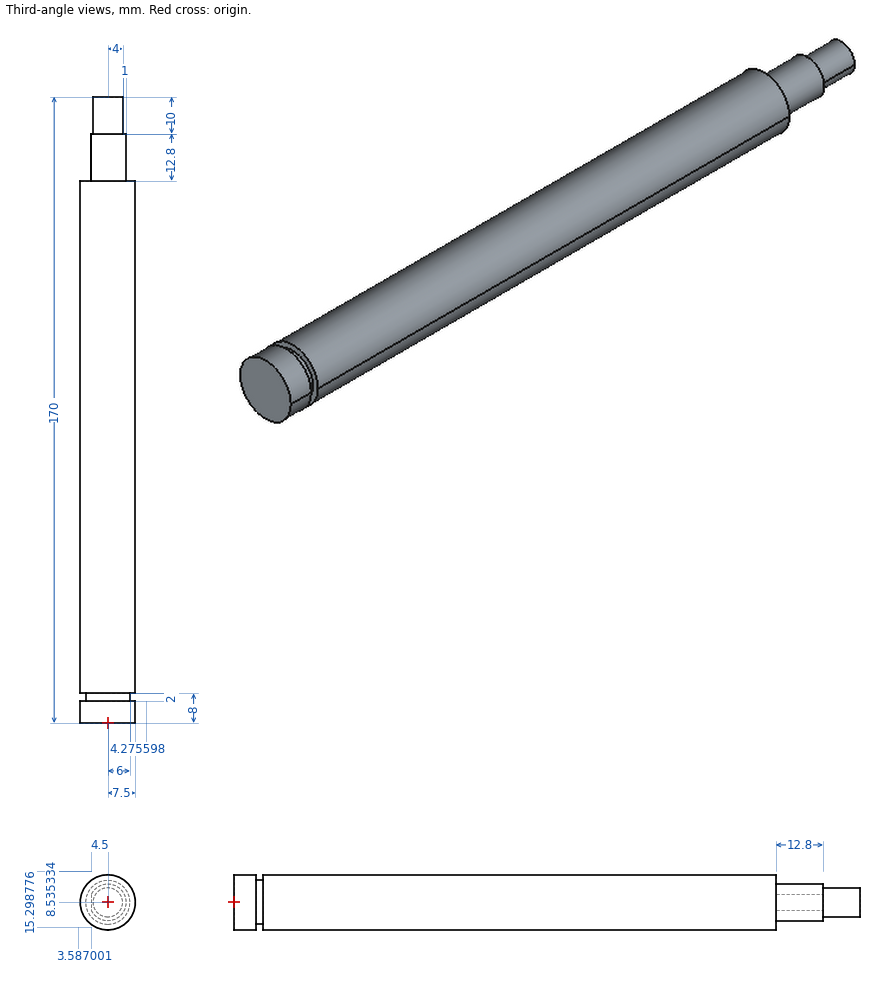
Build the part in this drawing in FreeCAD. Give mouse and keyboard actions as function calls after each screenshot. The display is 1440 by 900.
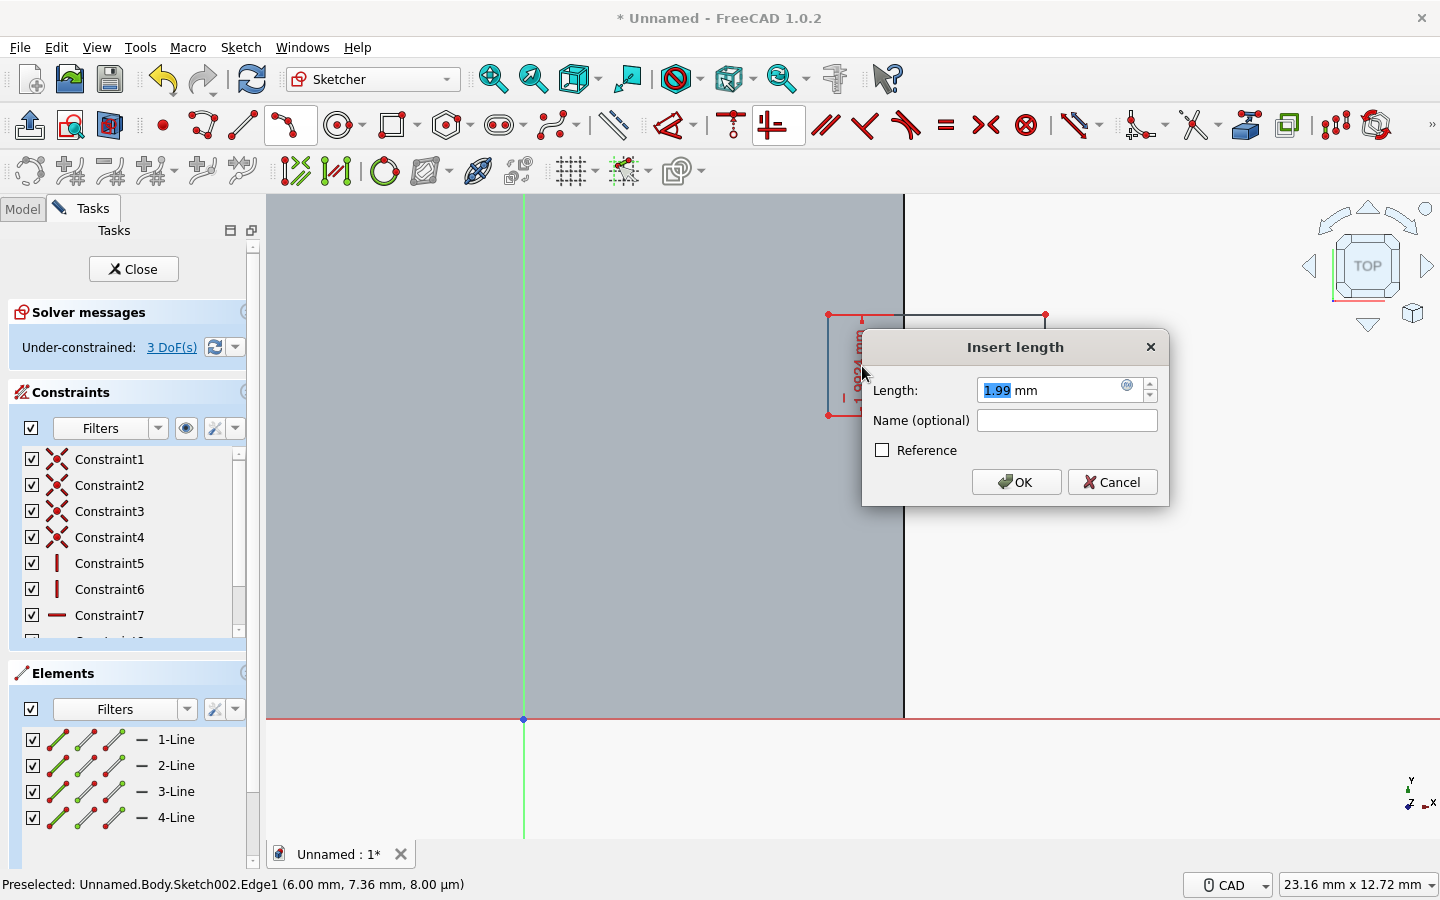
text(2)
key(Return)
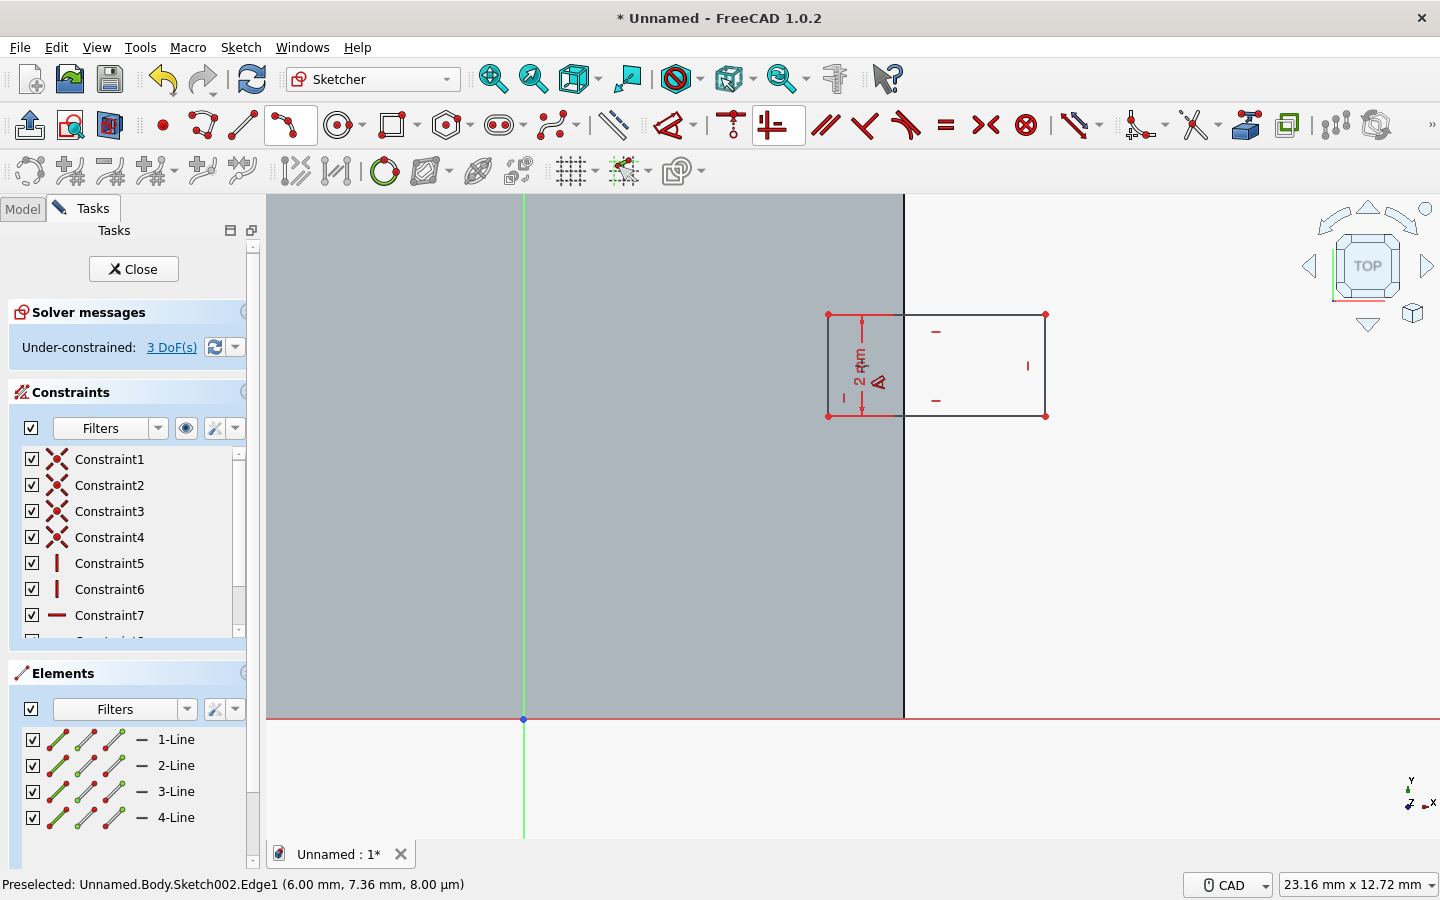
click(828, 315)
click(676, 753)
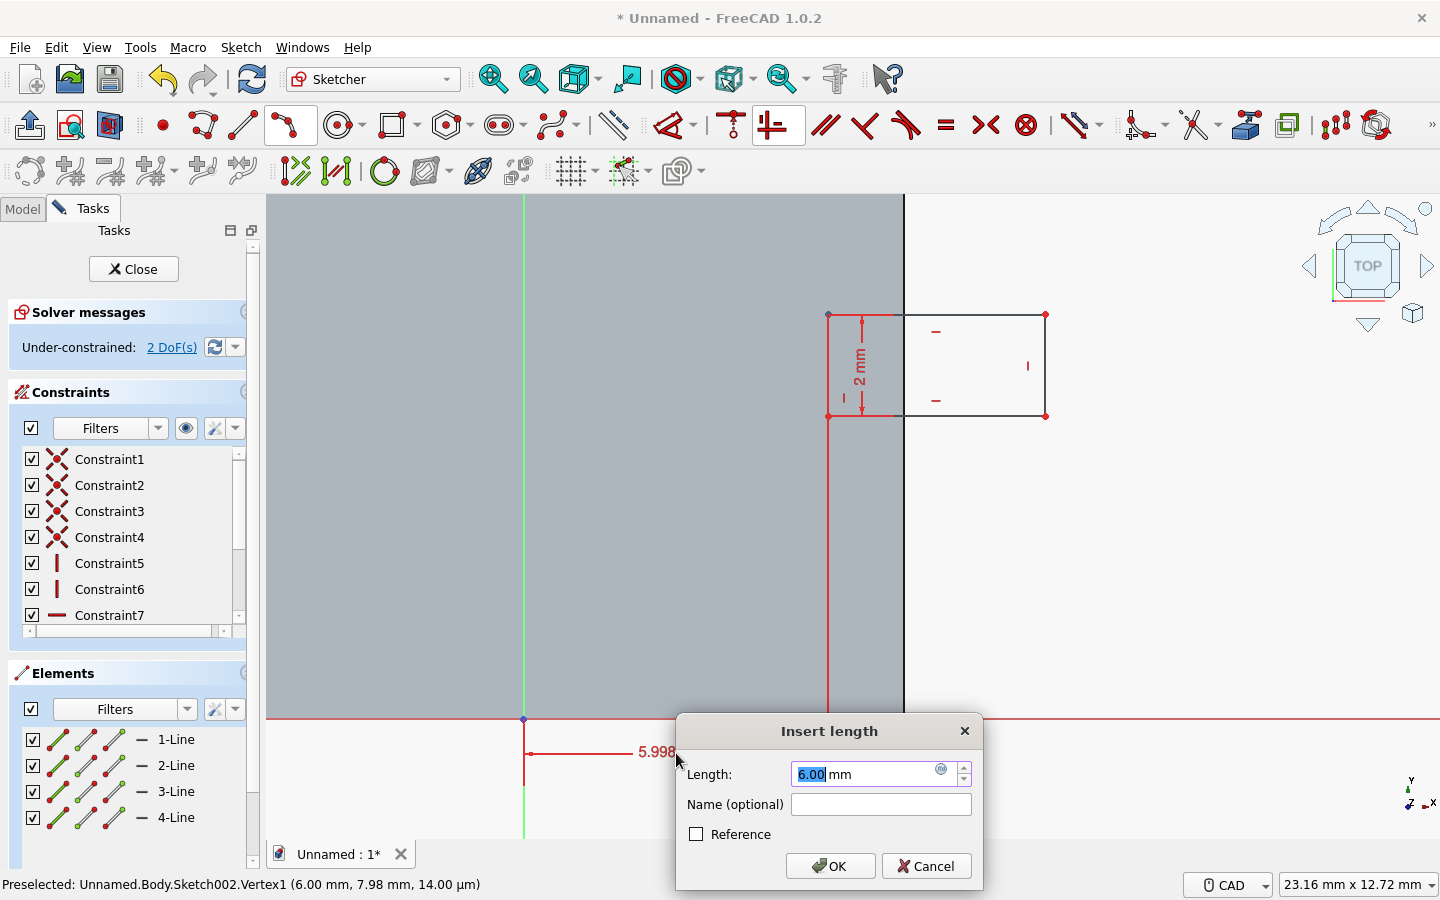
text(6)
key(Return)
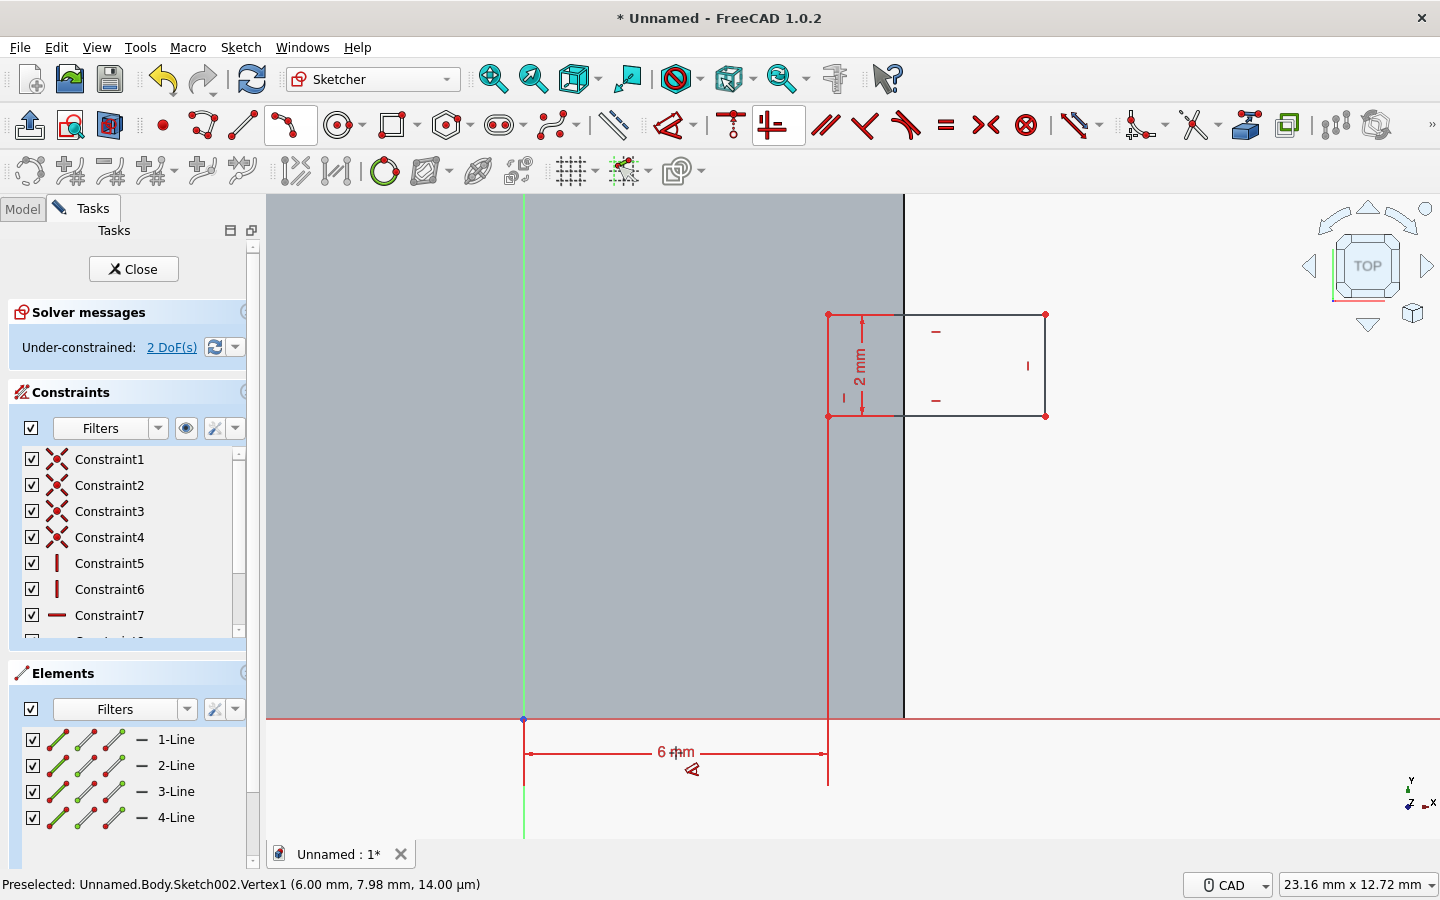
click(828, 315)
click(490, 517)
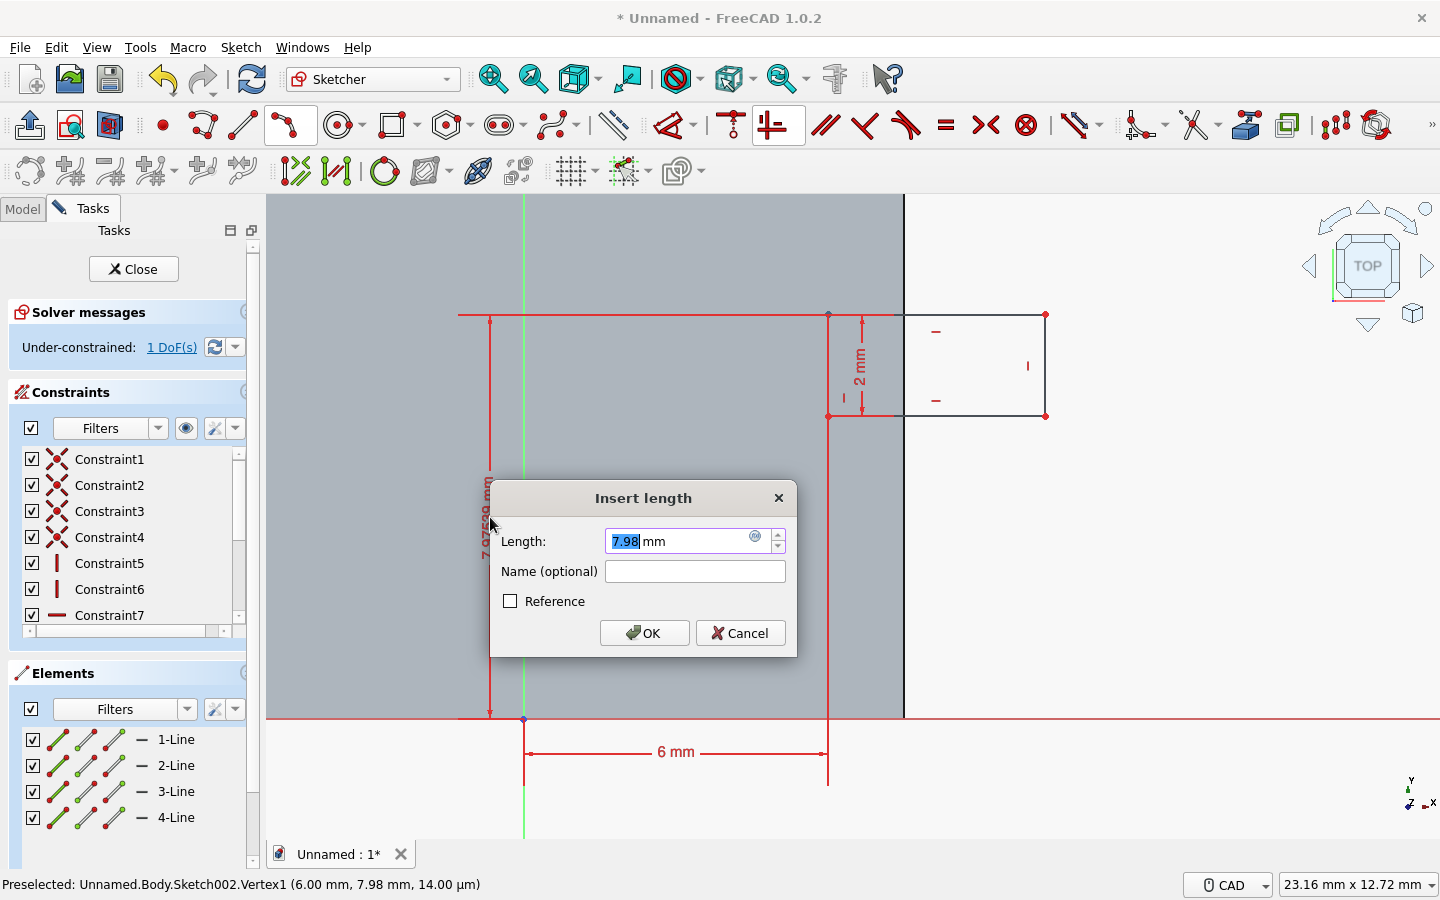
text(8)
key(Return)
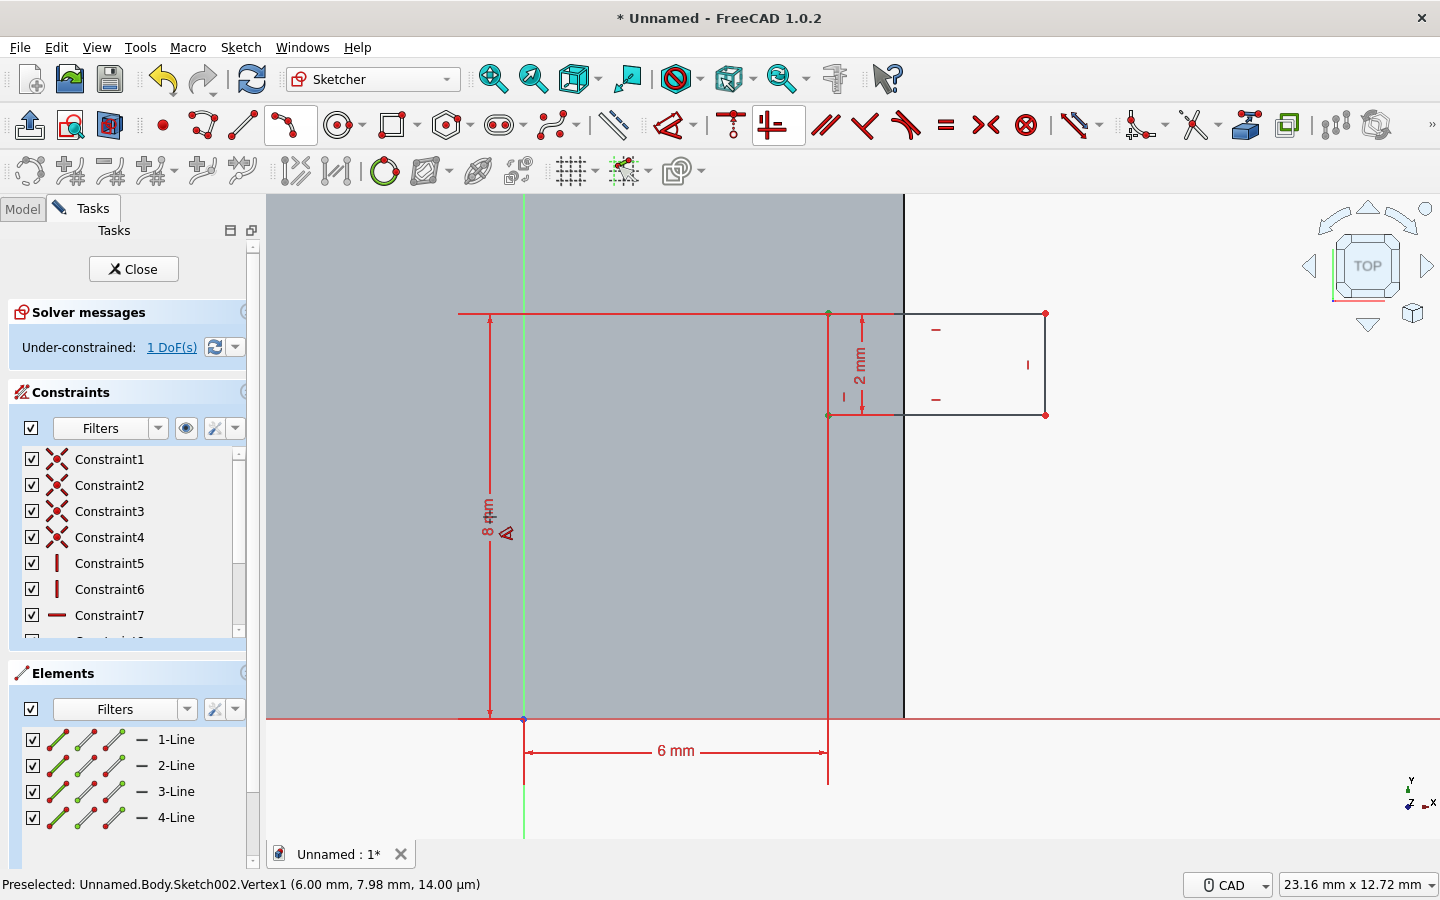
click(893, 415)
click(937, 381)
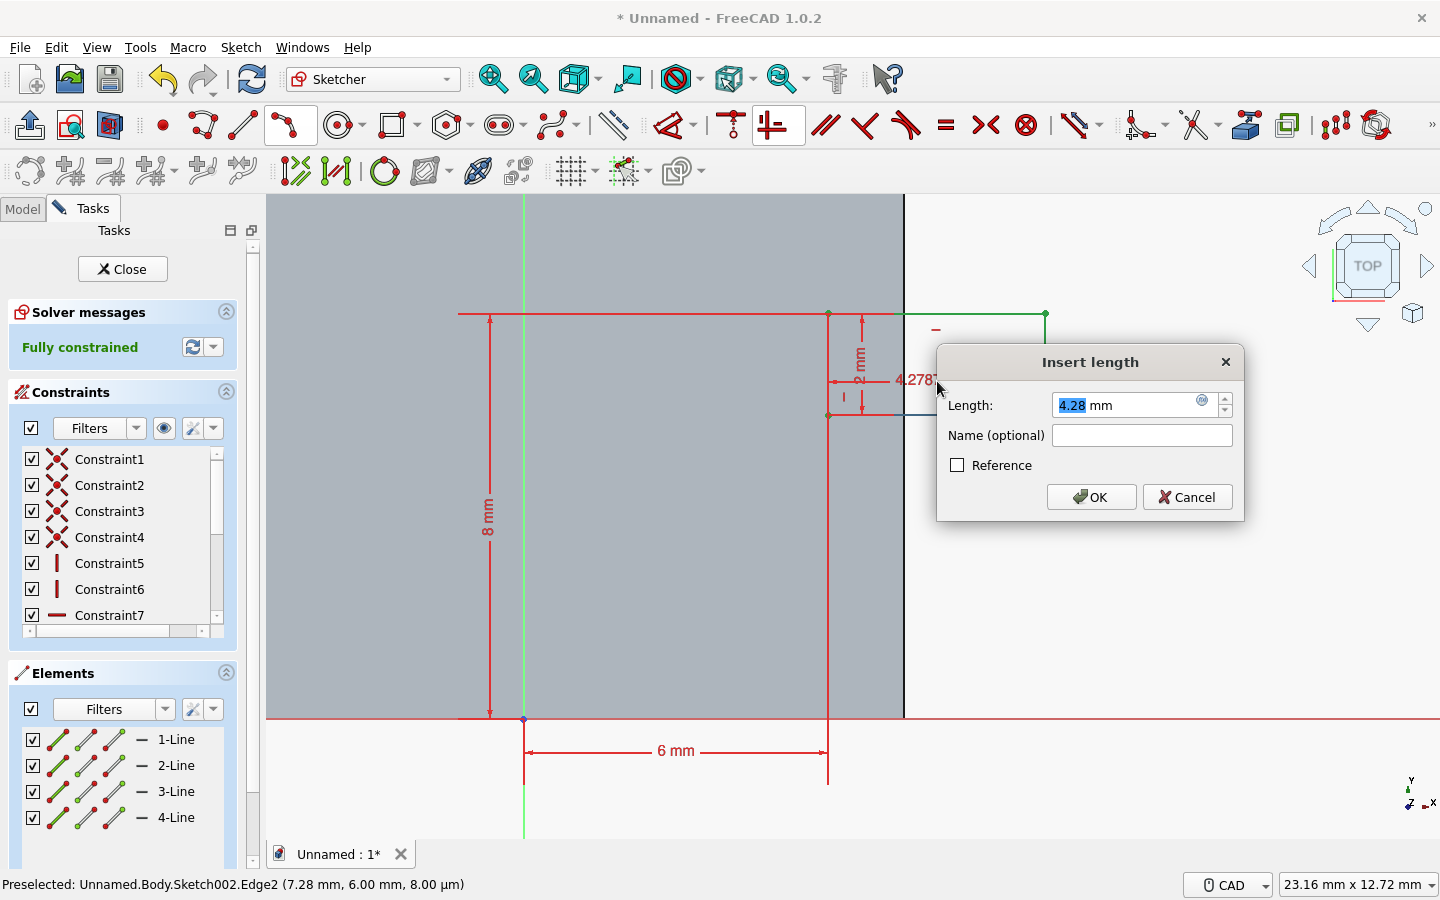
text(4.275598)
key(Return)
key(Escape)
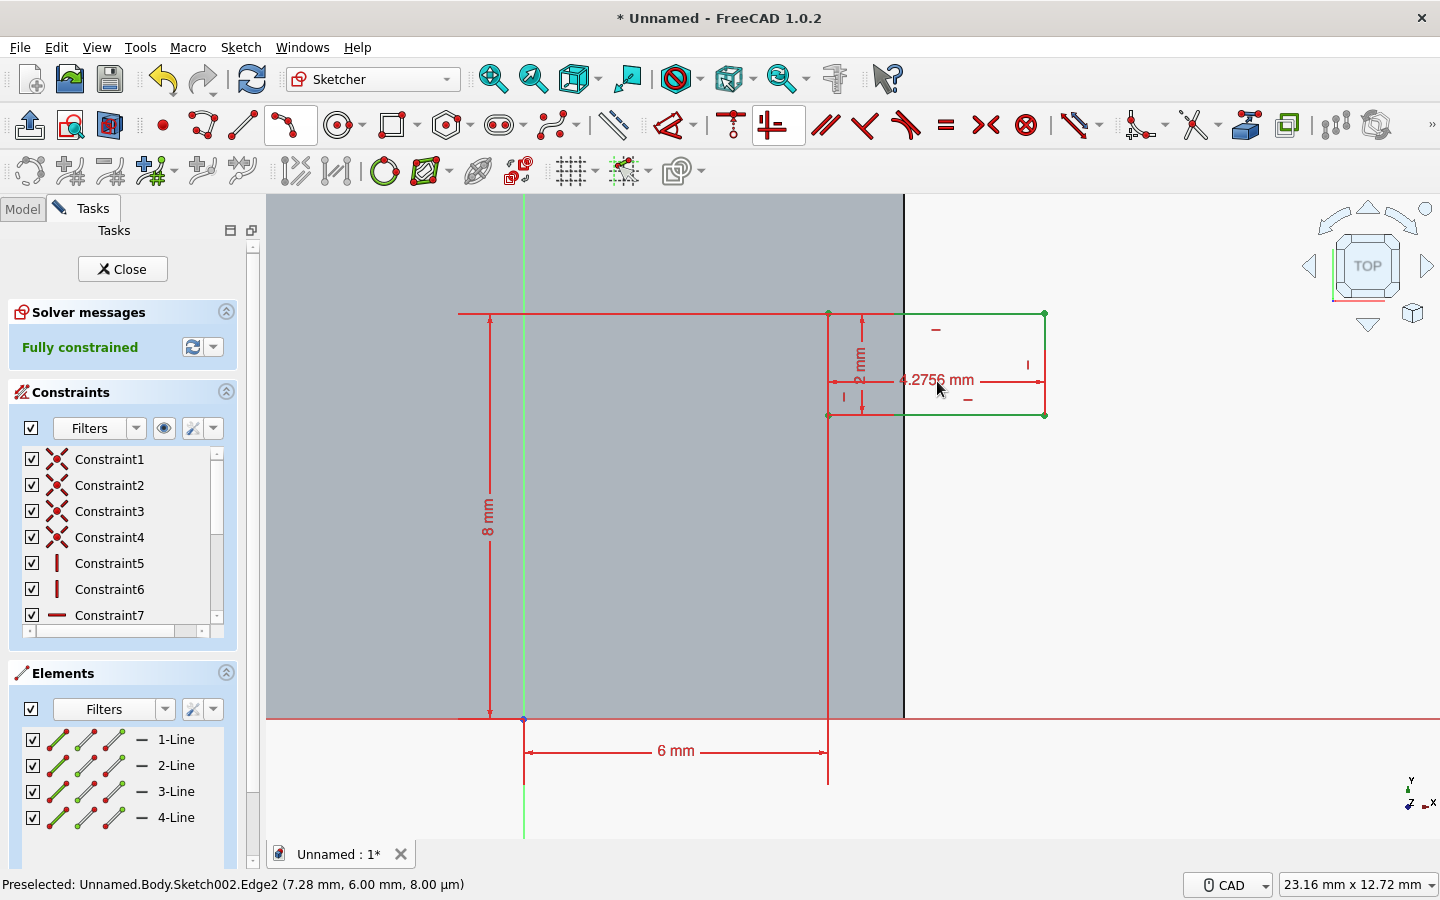
click(123, 269)